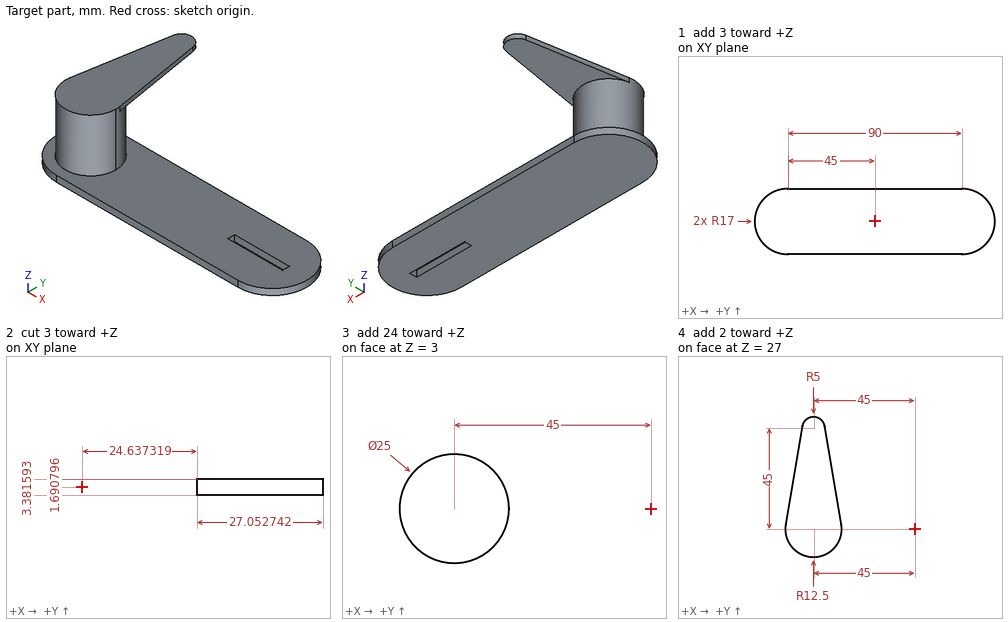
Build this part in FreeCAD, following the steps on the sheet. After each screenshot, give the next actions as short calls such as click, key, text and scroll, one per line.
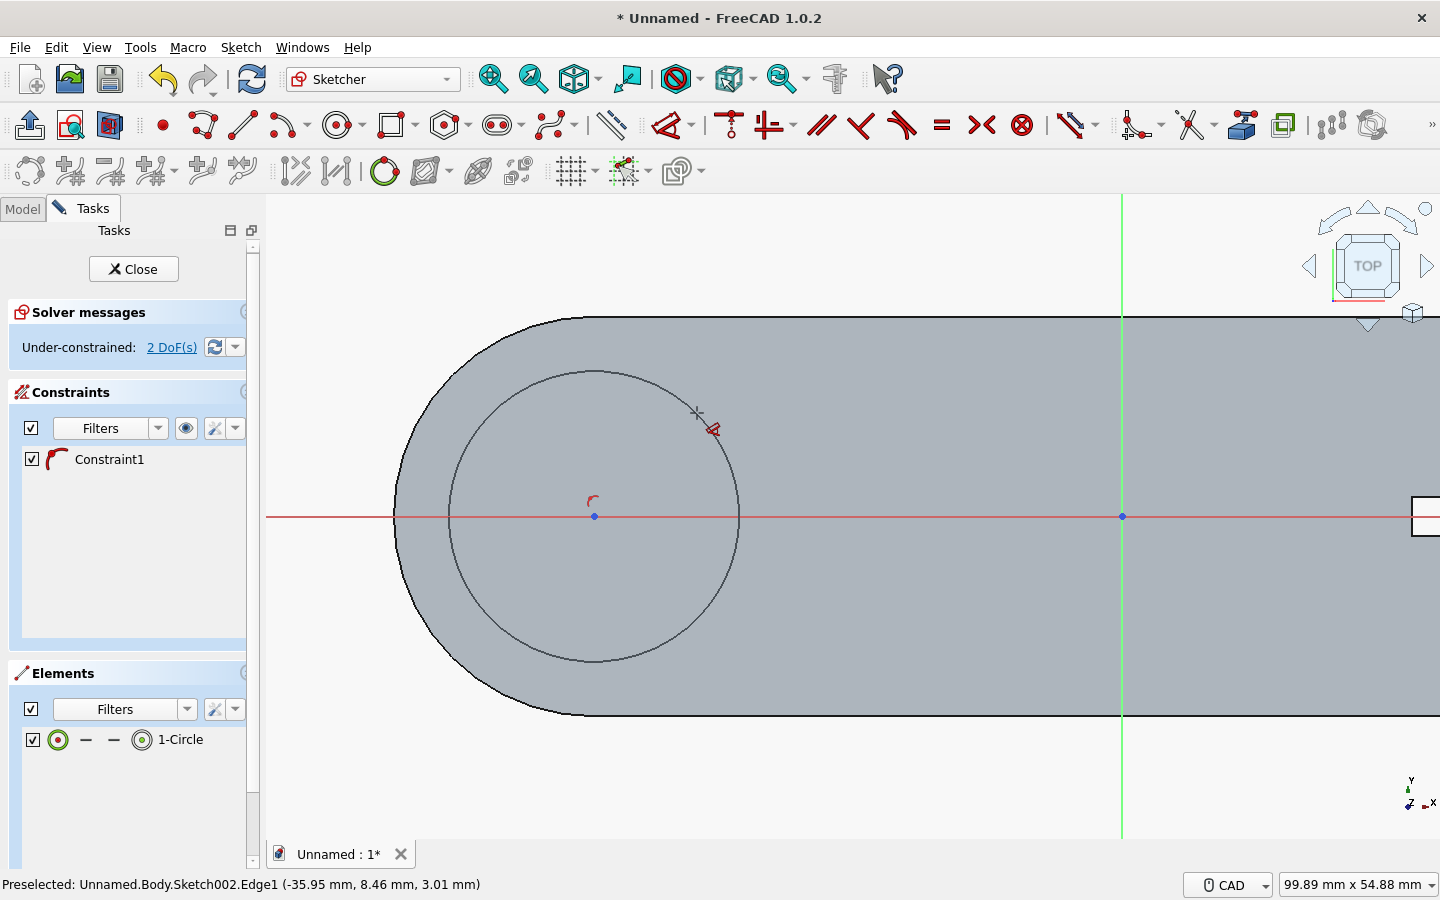
click(696, 413)
click(718, 390)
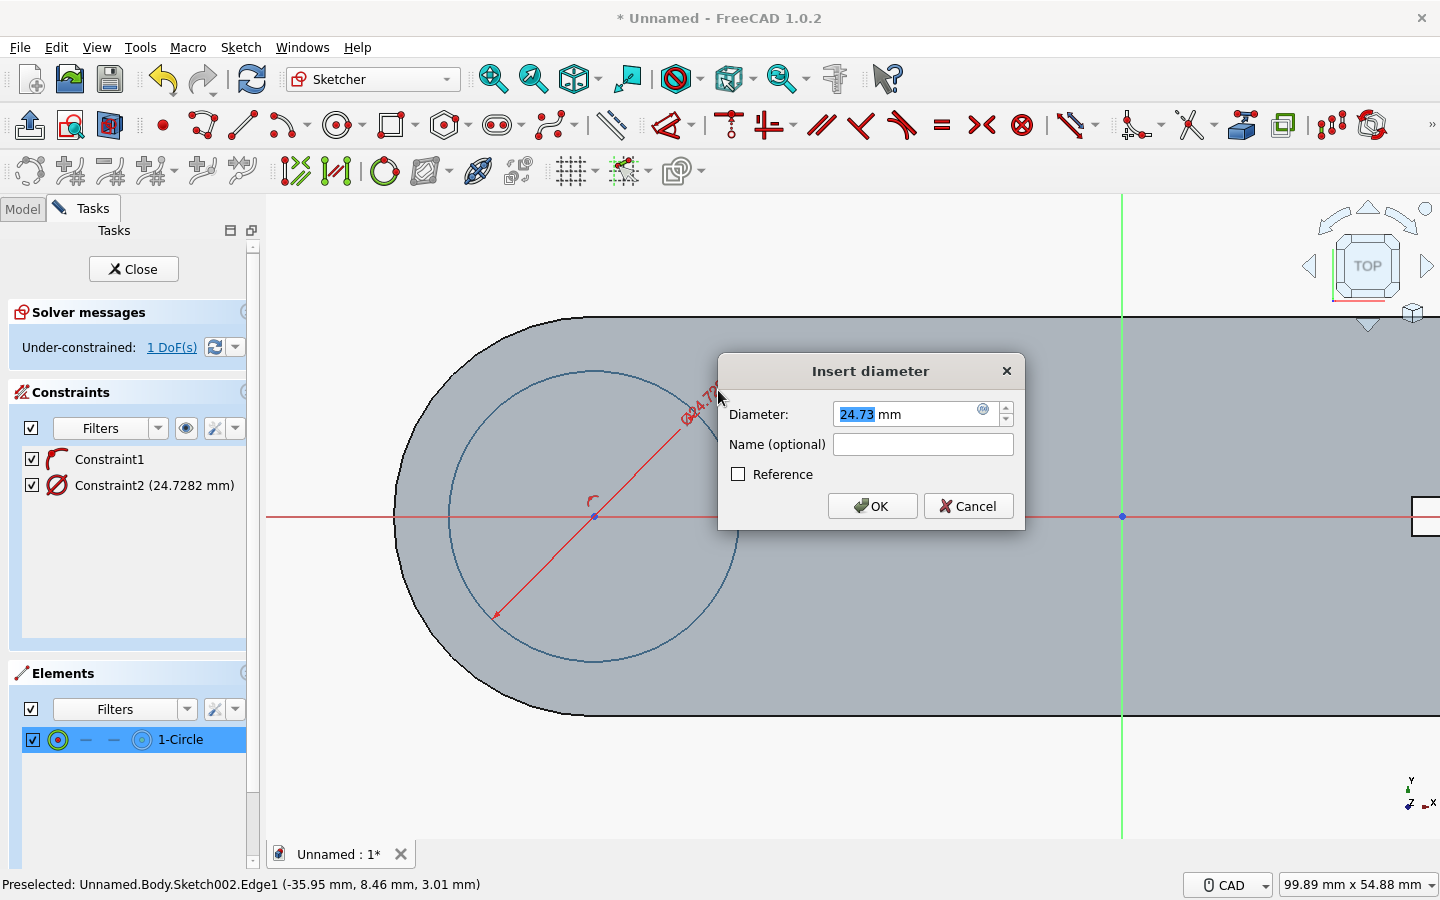
text(25)
key(Return)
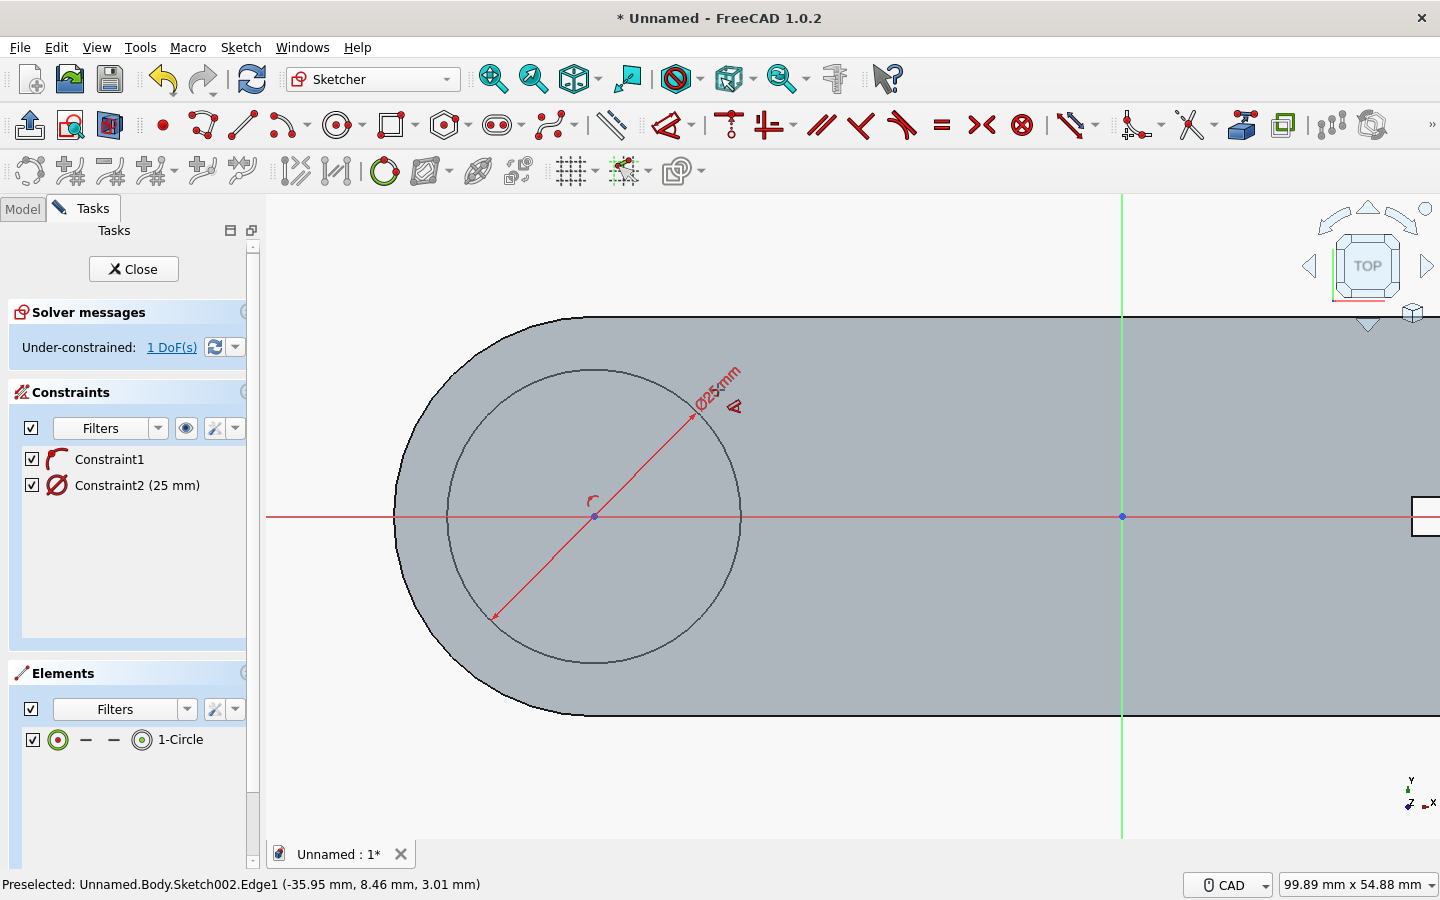
click(594, 516)
click(858, 550)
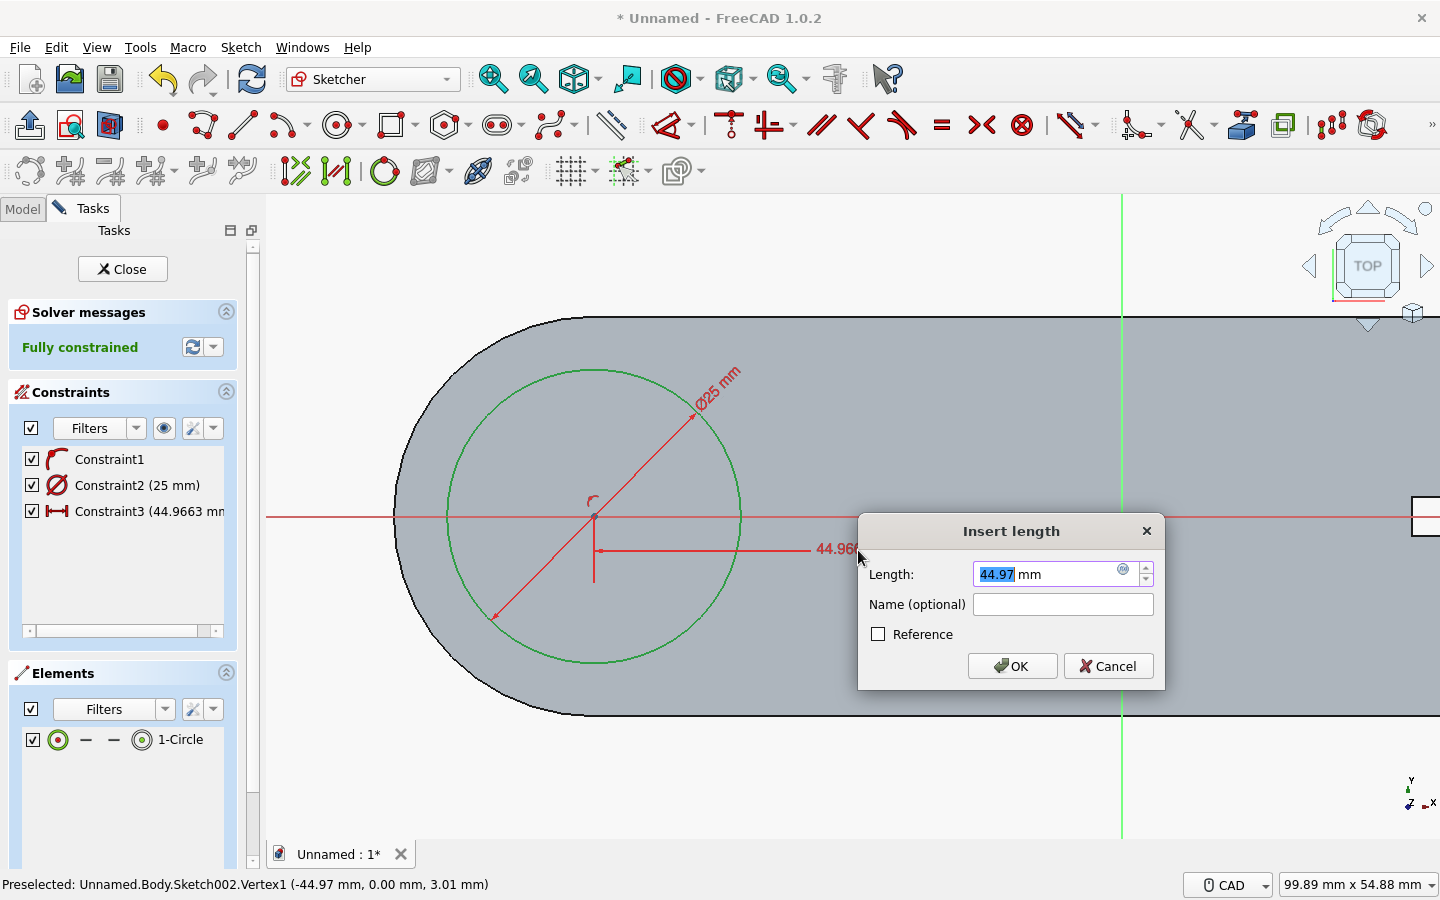
text(45)
key(Return)
key(Escape)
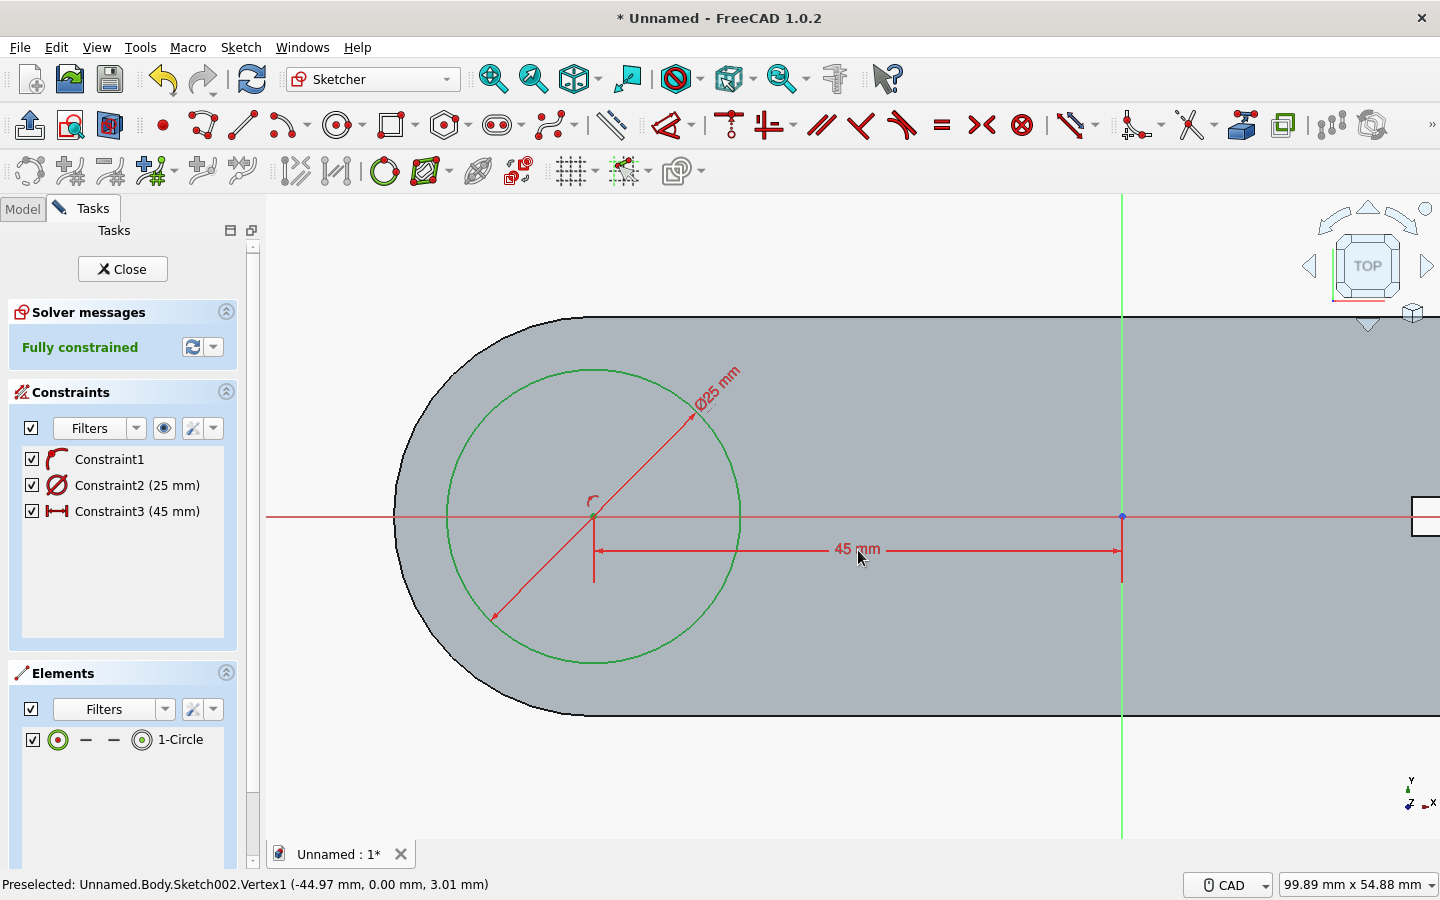
click(123, 269)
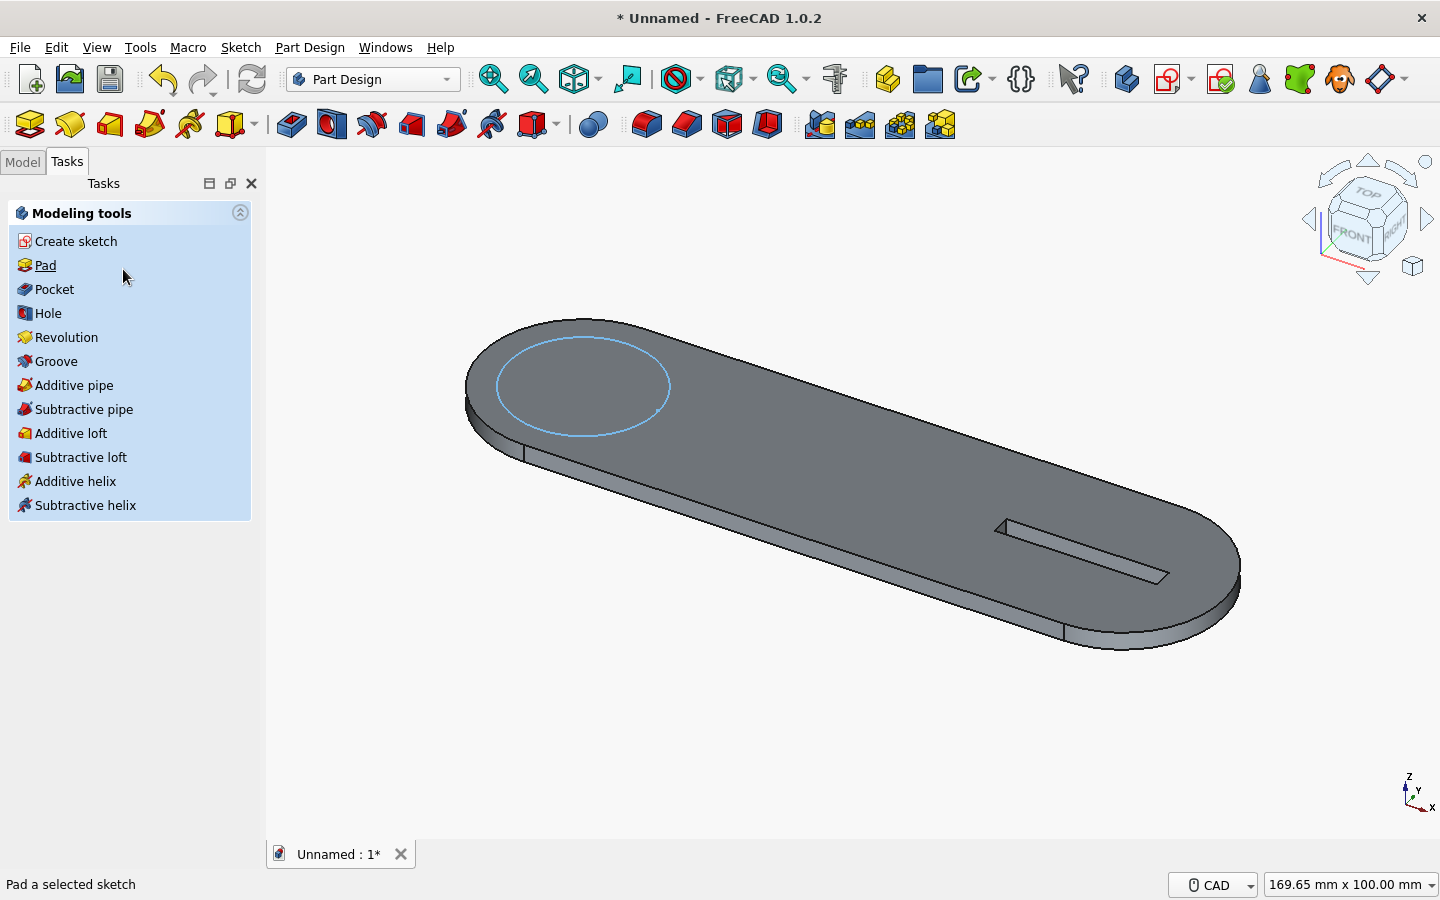
click(30, 124)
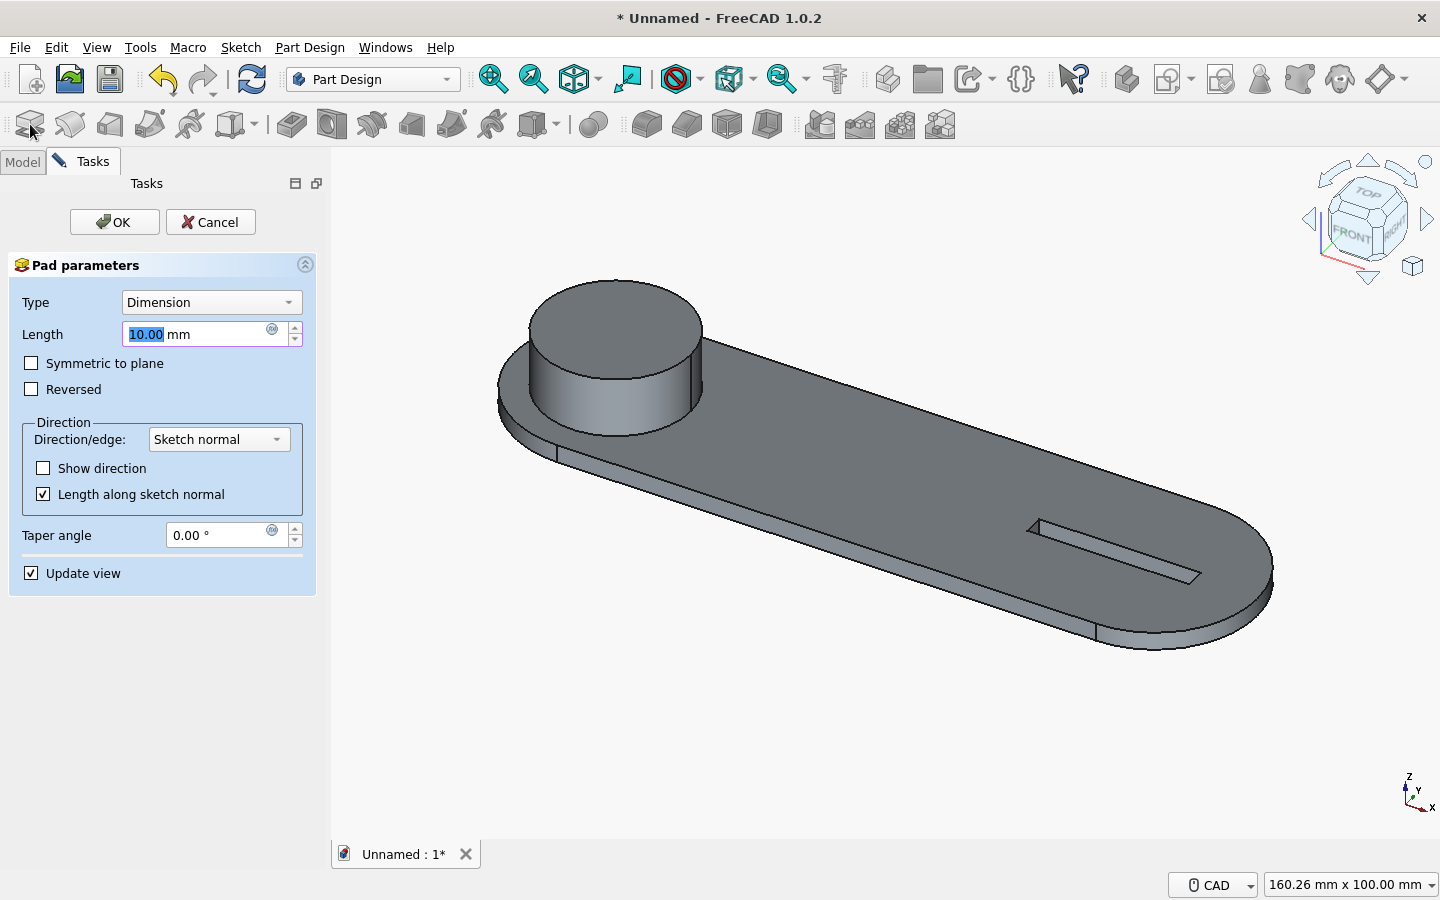
text(24)
key(Tab)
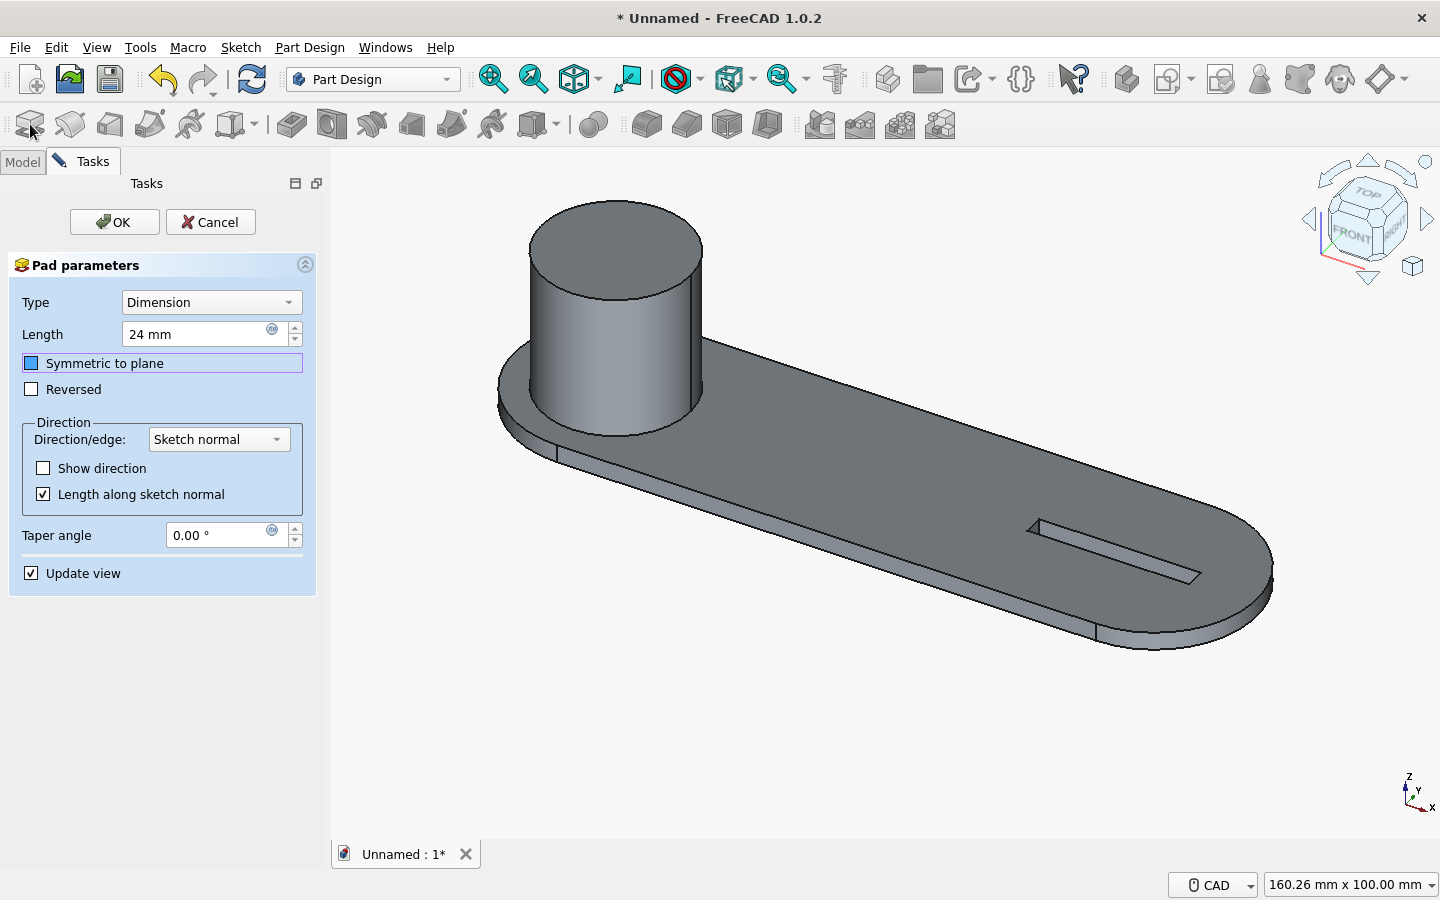
click(115, 222)